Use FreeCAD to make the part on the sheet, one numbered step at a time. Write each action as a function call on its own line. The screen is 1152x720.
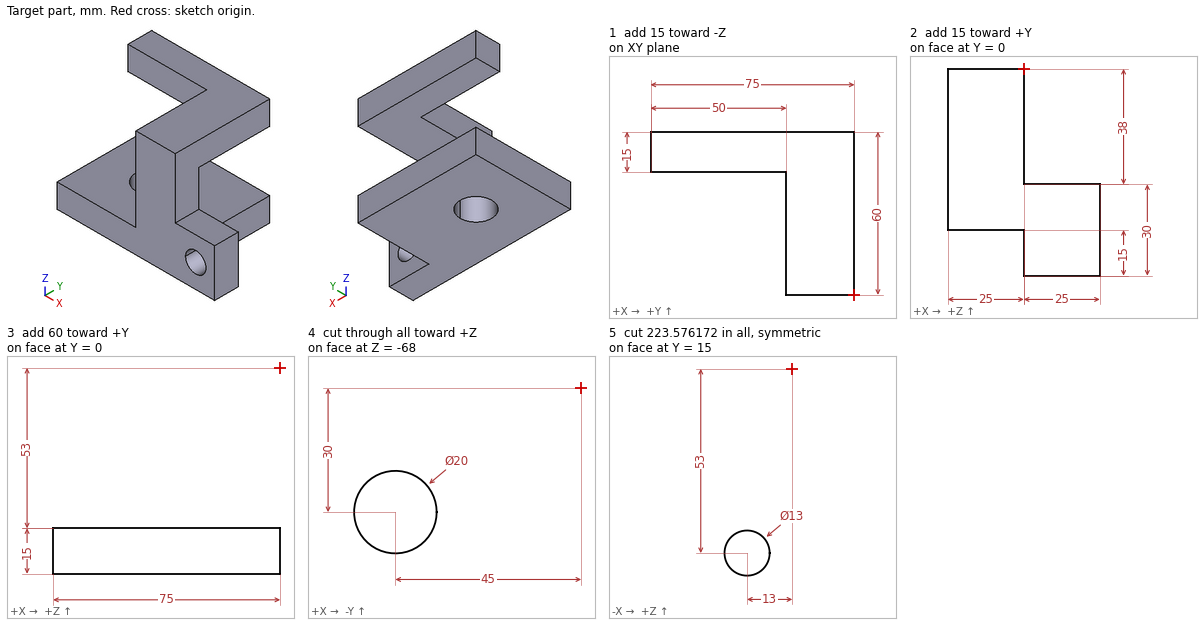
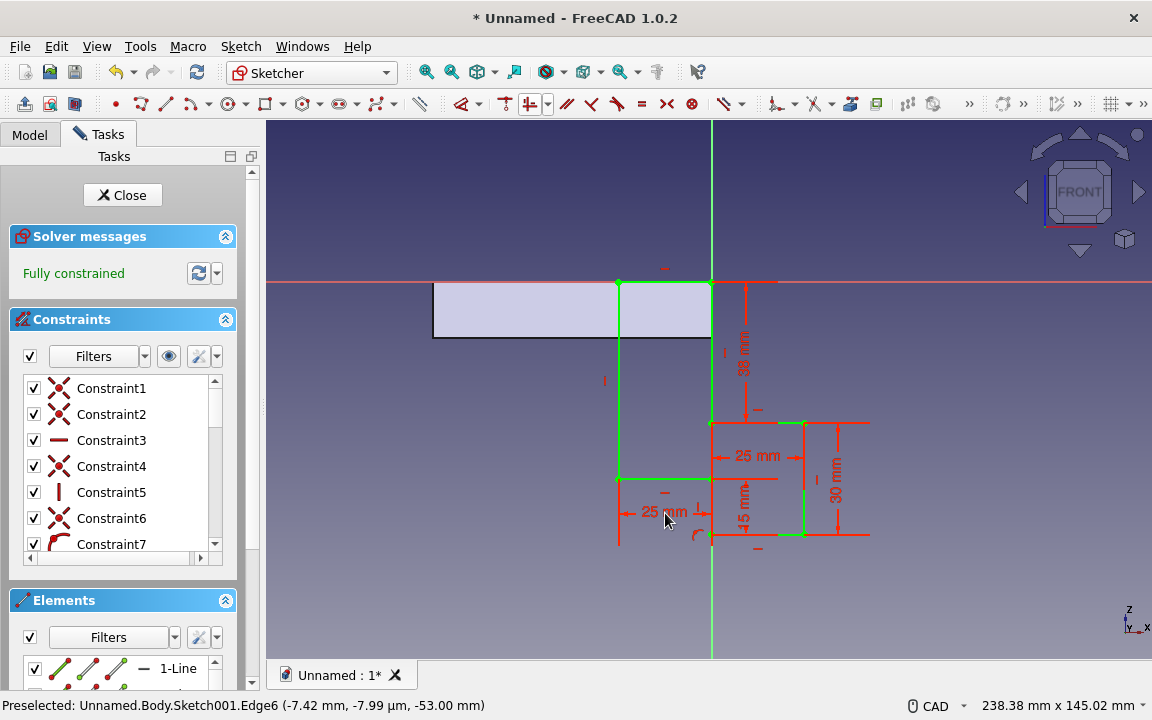
click(123, 195)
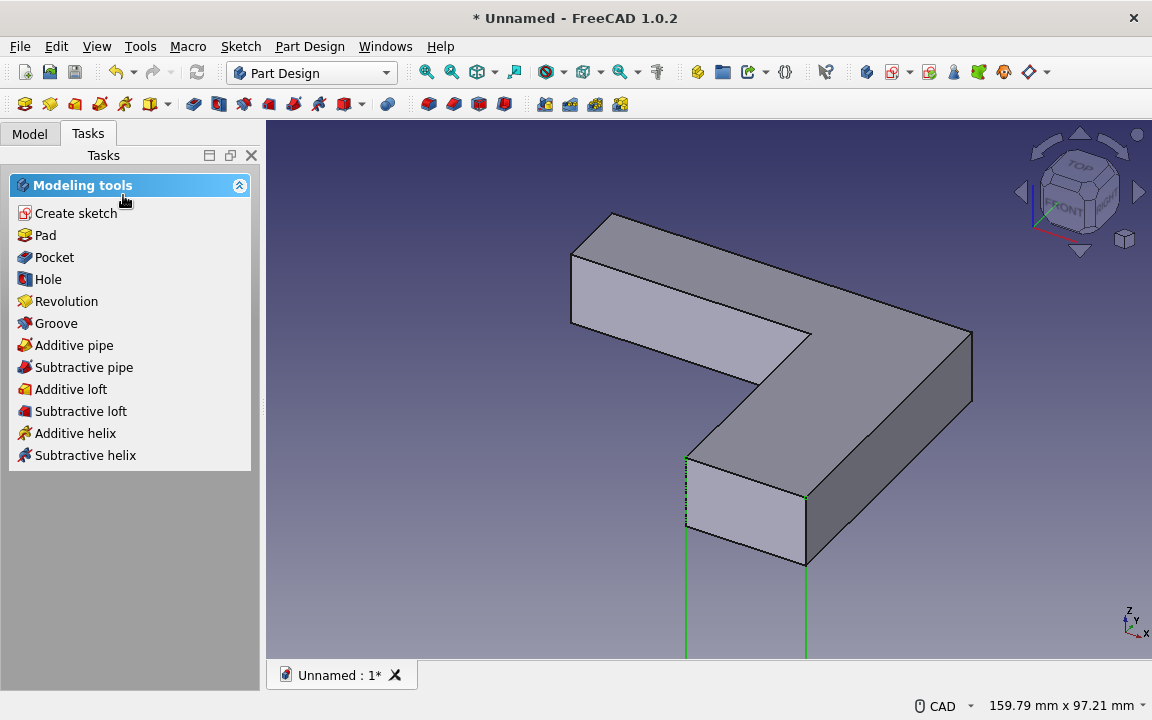
click(25, 104)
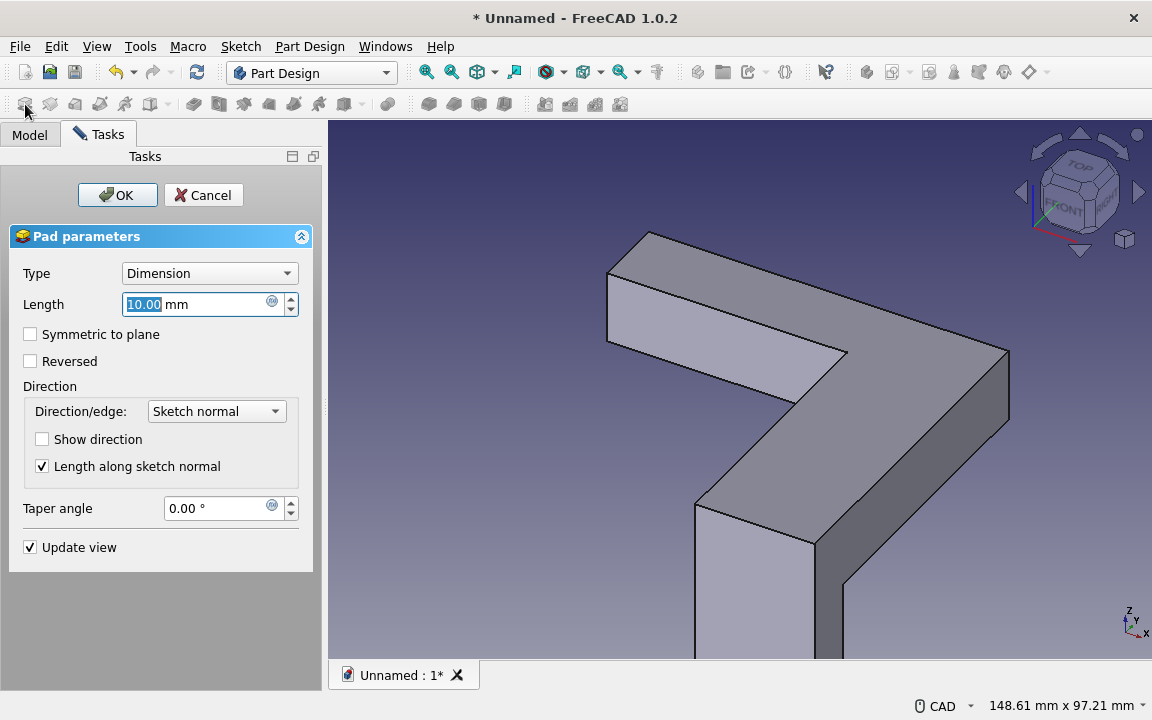
text(15)
key(Tab)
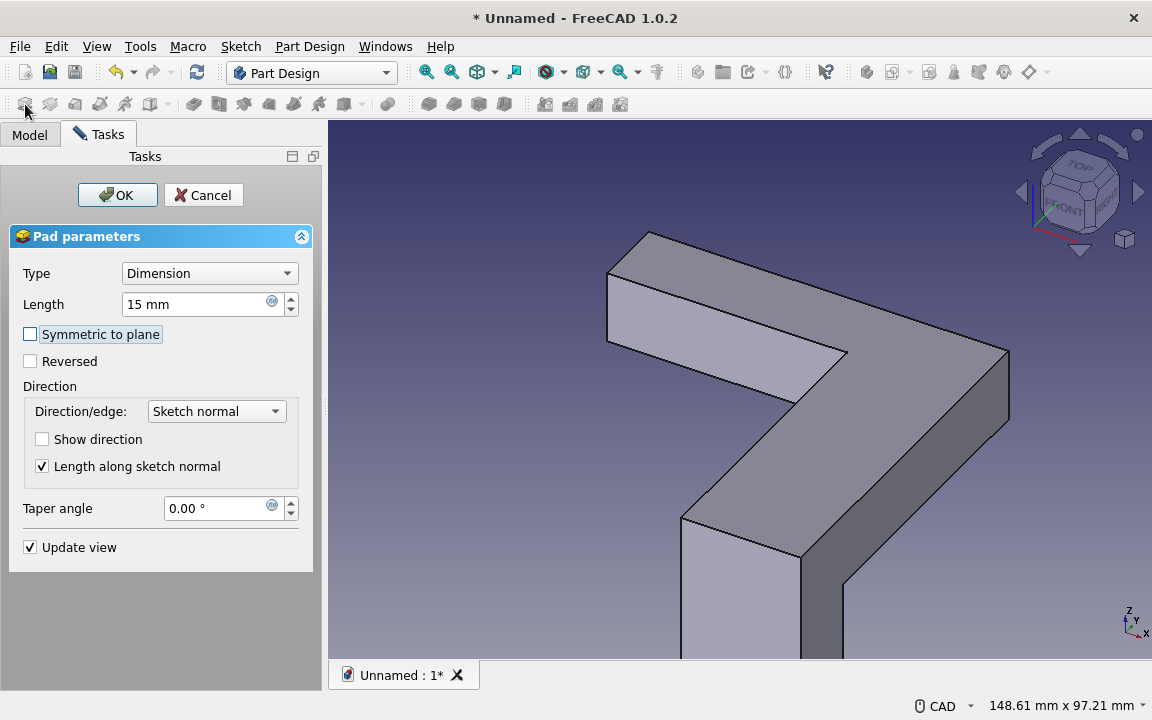
click(31, 361)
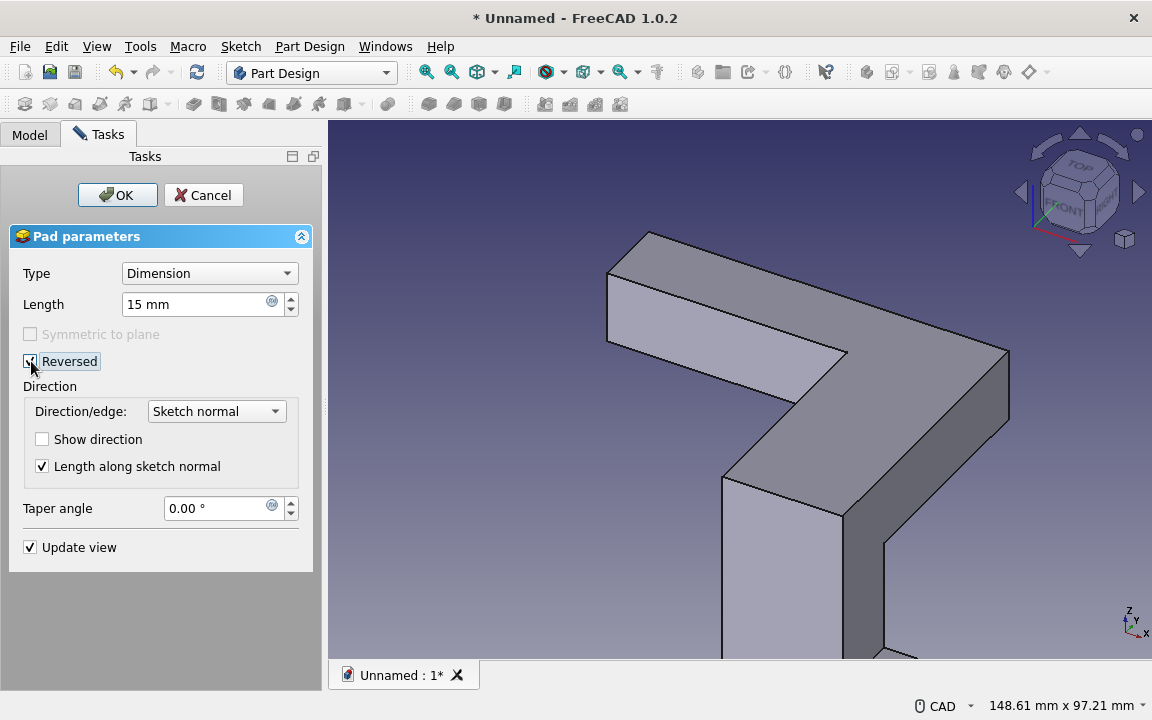
click(118, 195)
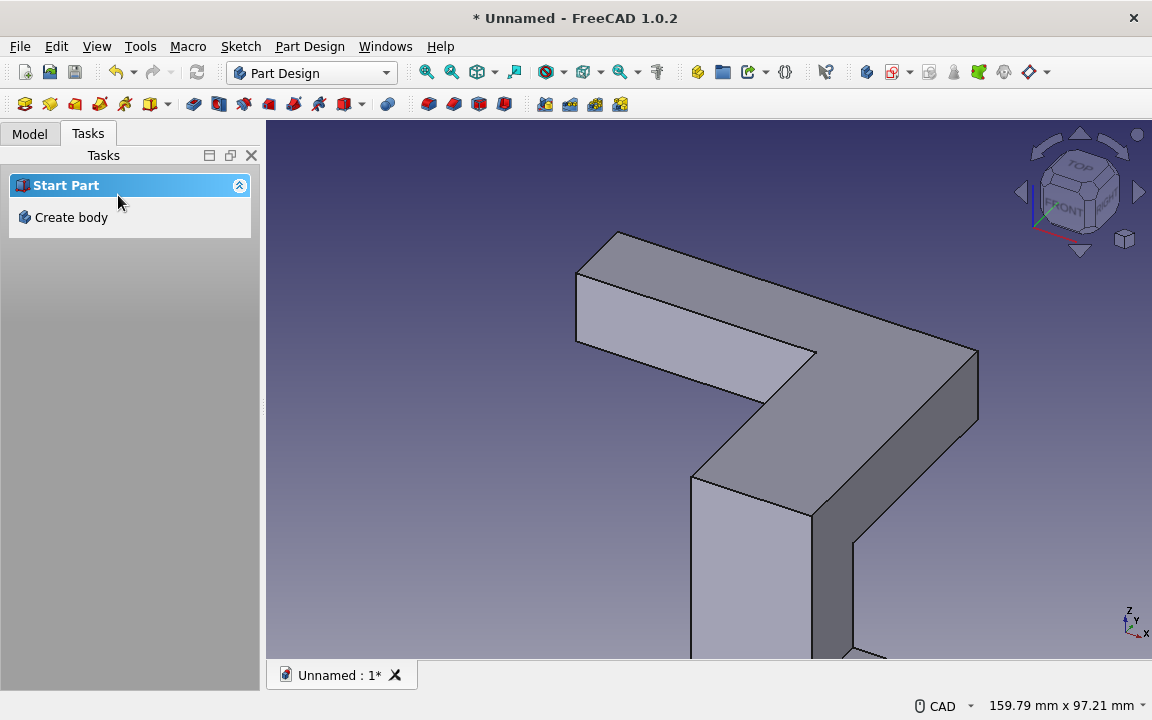
key(v)
key(f)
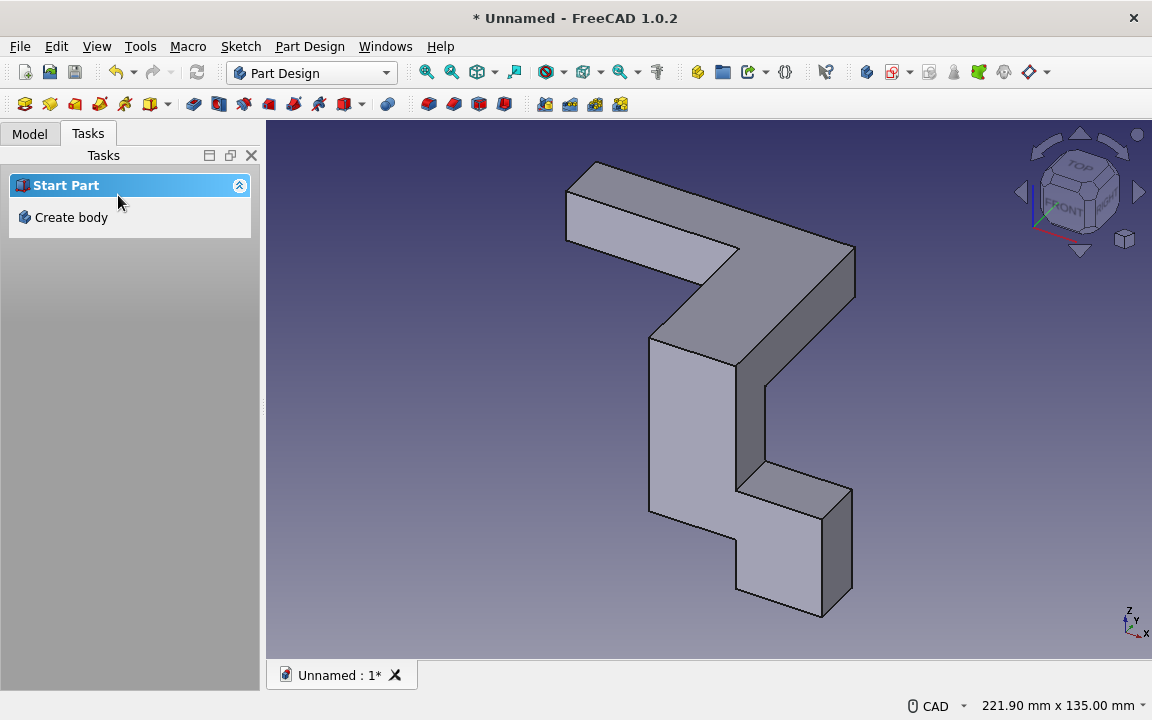
click(785, 557)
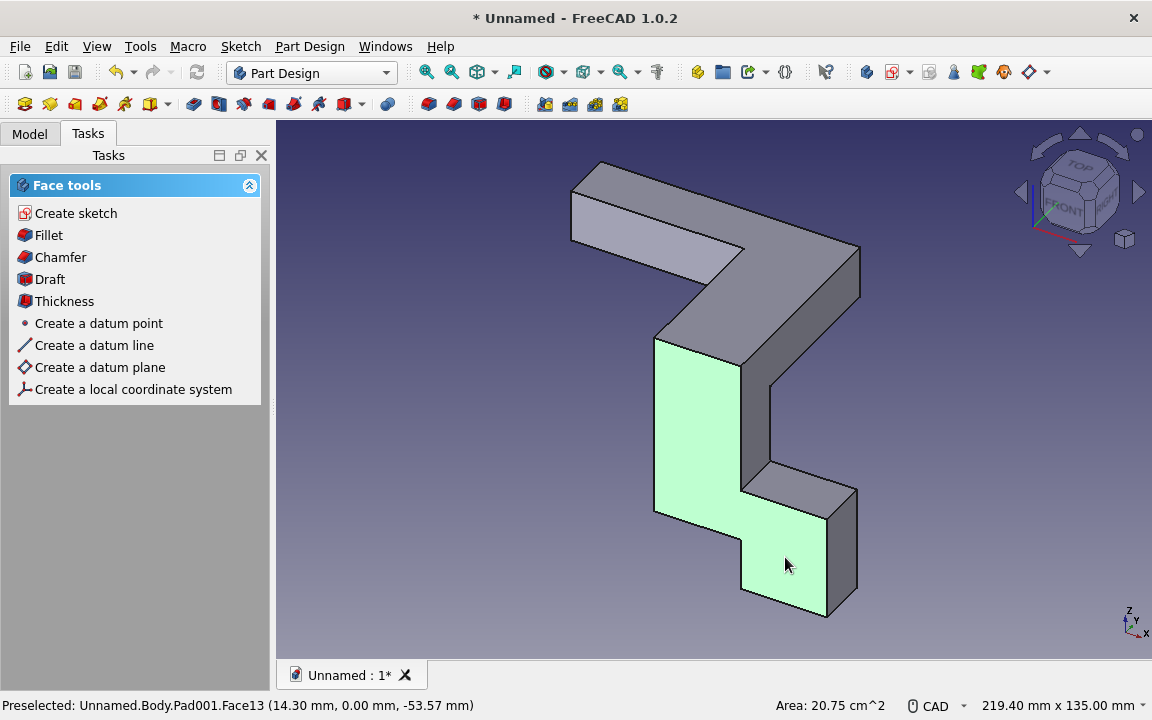
click(892, 72)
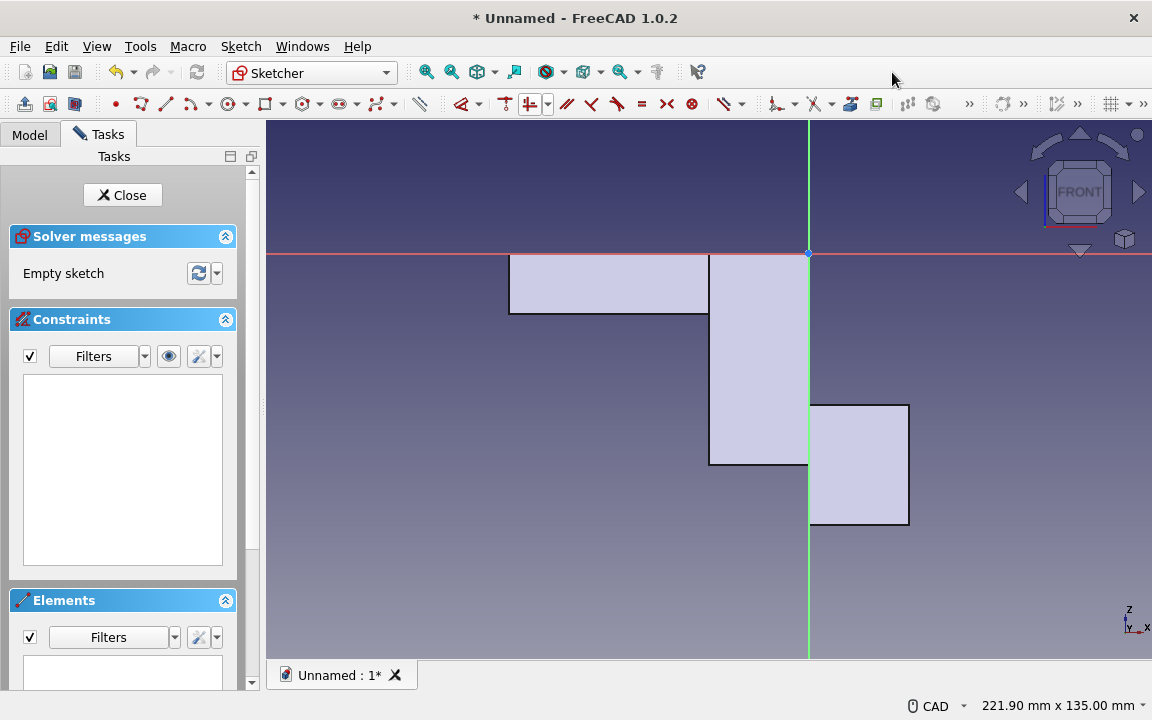
click(264, 104)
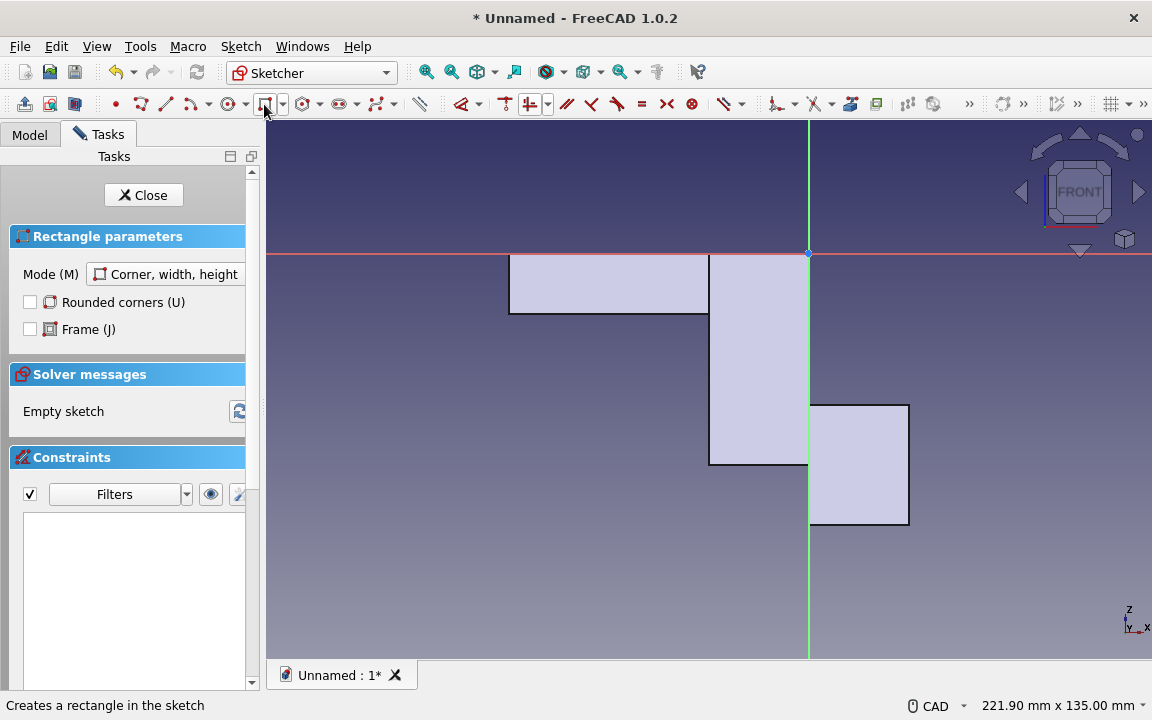
click(509, 465)
click(809, 525)
key(Escape)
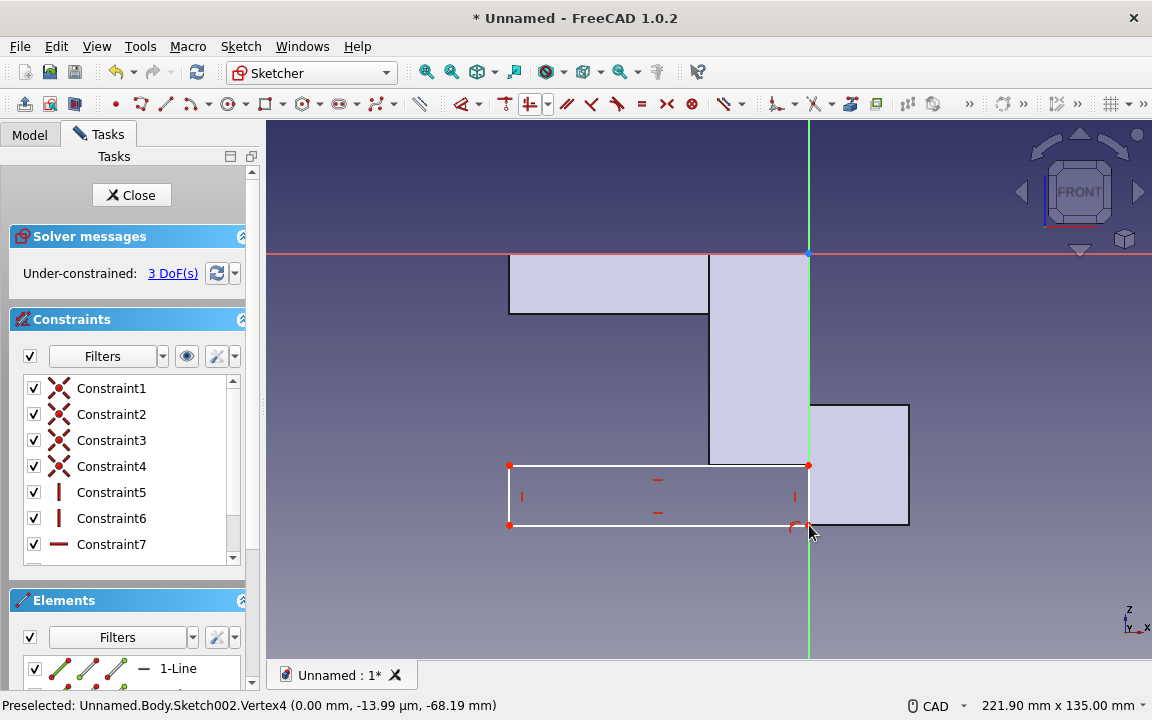
key(d)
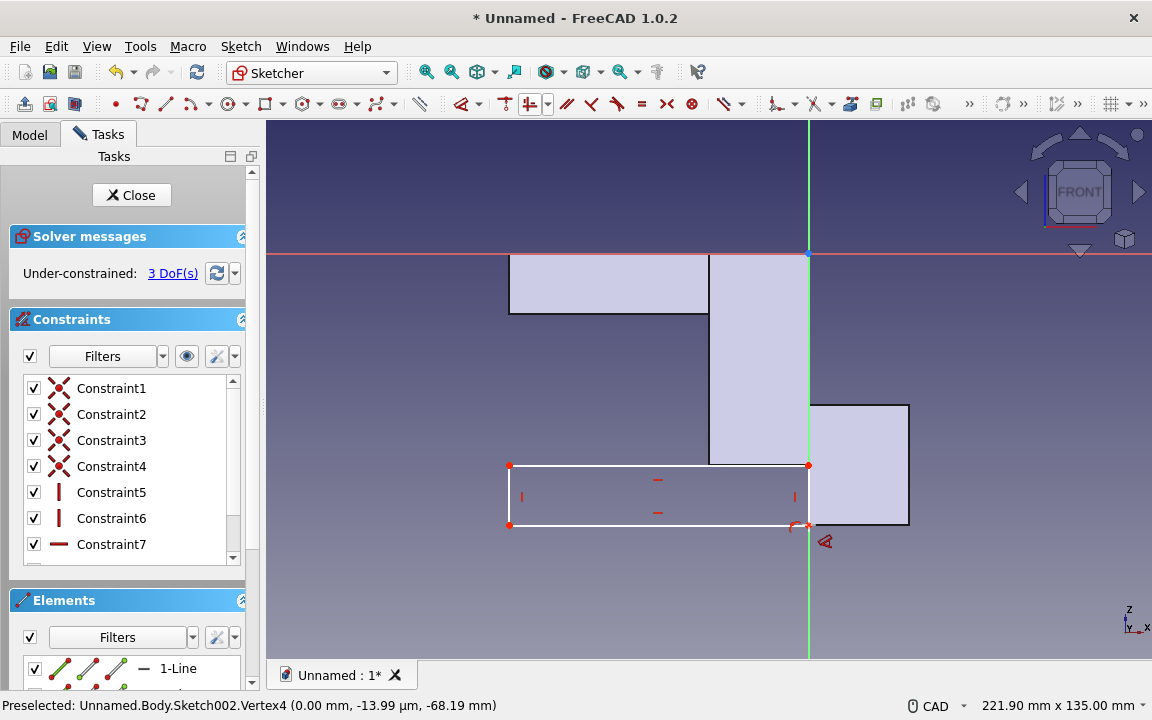
click(509, 484)
click(475, 496)